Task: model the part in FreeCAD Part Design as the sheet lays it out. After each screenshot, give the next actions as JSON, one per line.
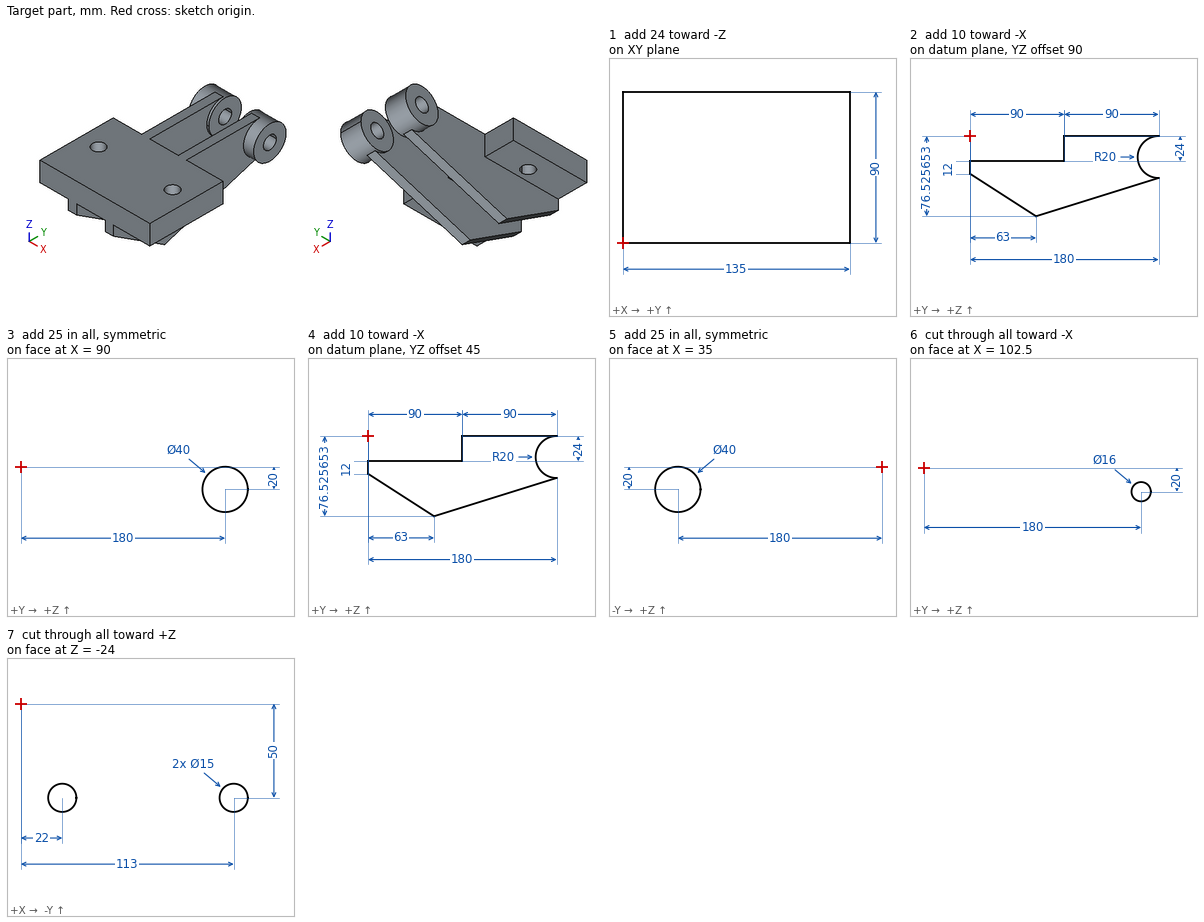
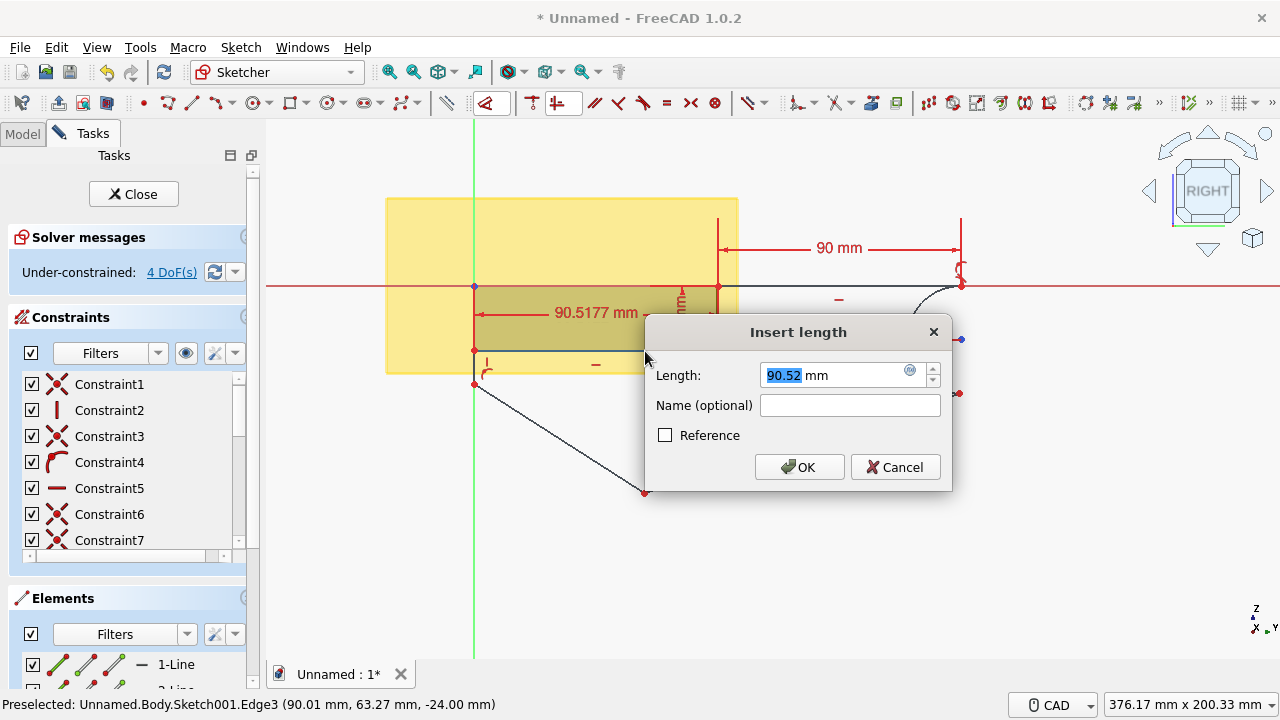
{"action": "type", "text": "90"}
{"action": "key", "text": "Return"}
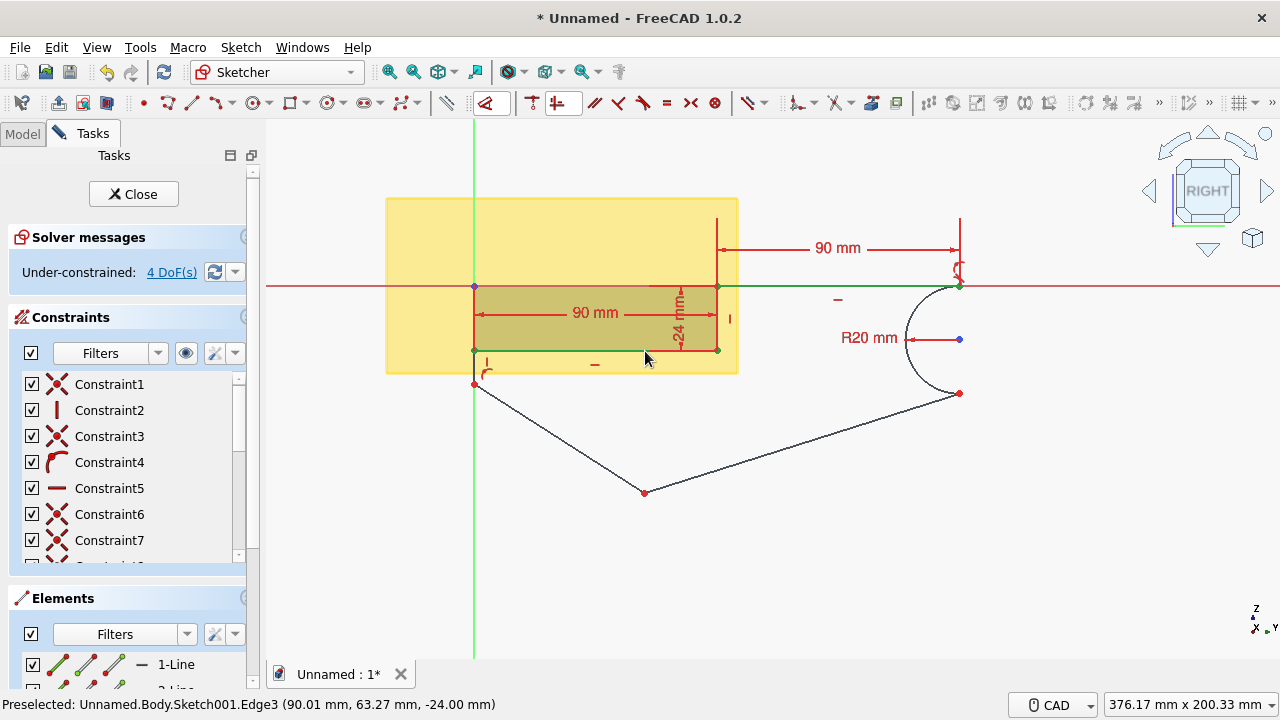
{"action": "scroll", "coordinate": [474, 361], "scroll_direction": "up", "scroll_amount": 2}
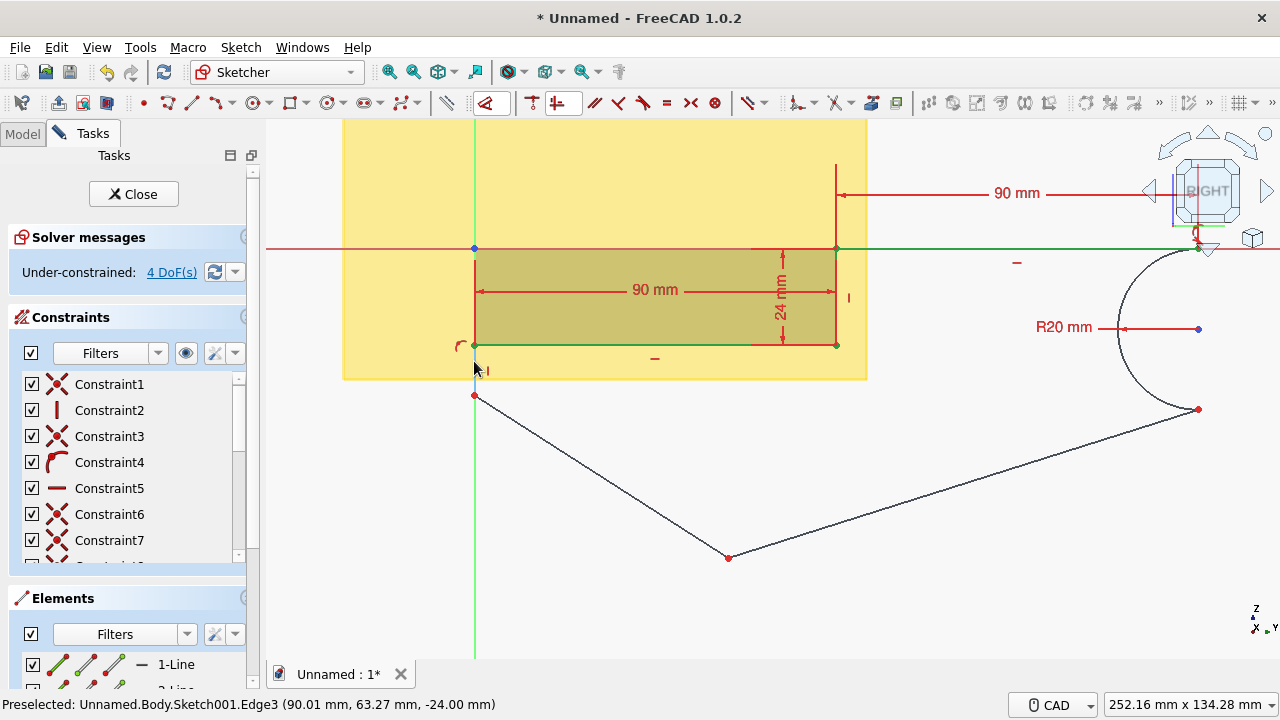
{"action": "left_click", "coordinate": [475, 360]}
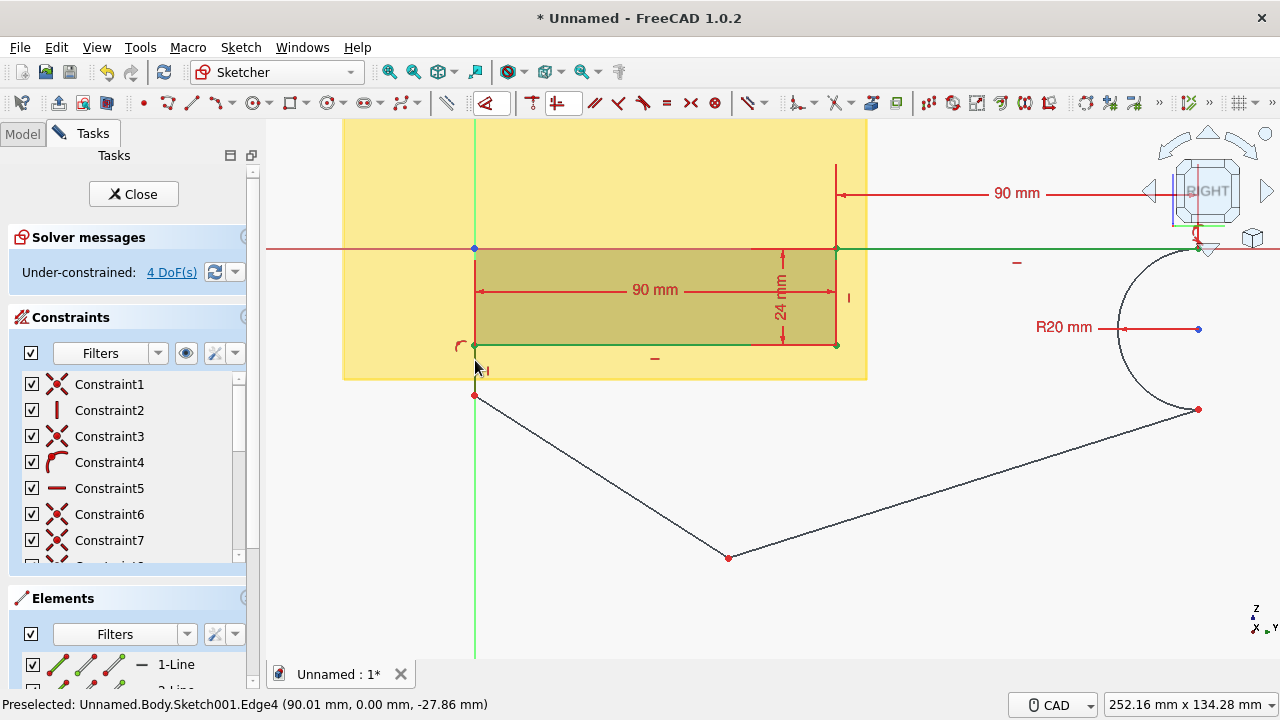
{"action": "key", "text": "i"}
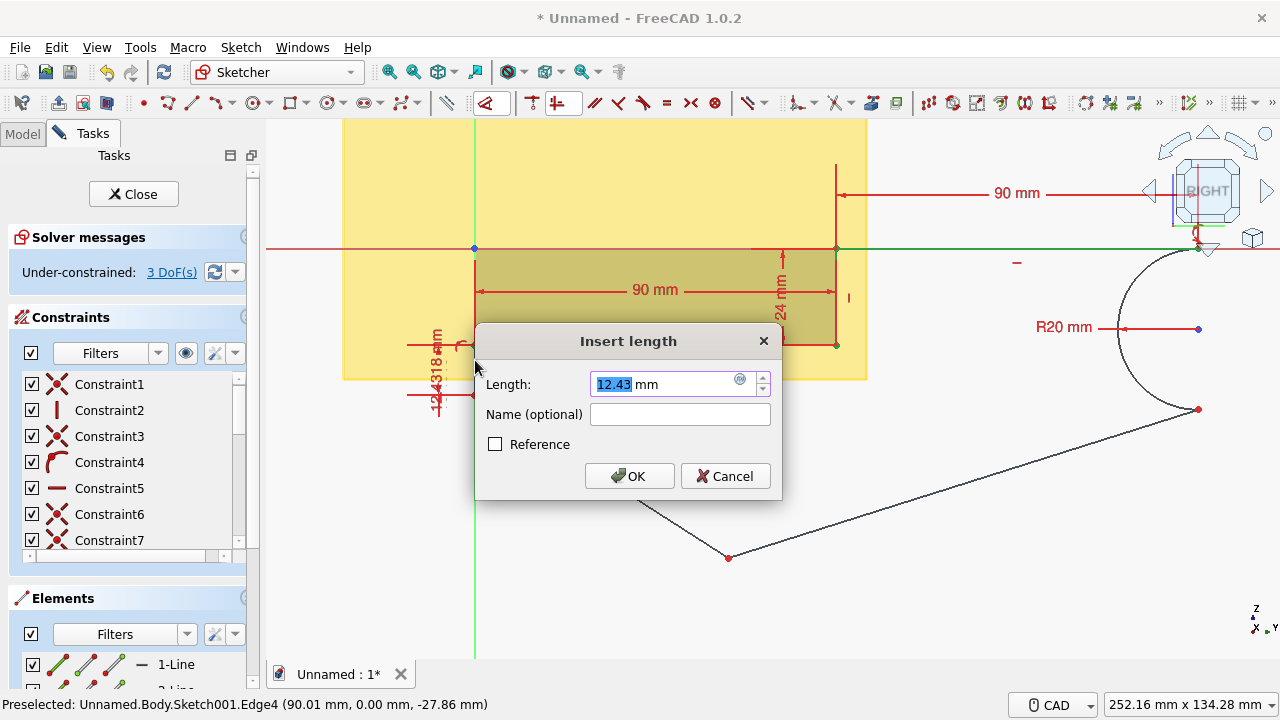
{"action": "type", "text": "12"}
{"action": "key", "text": "Return"}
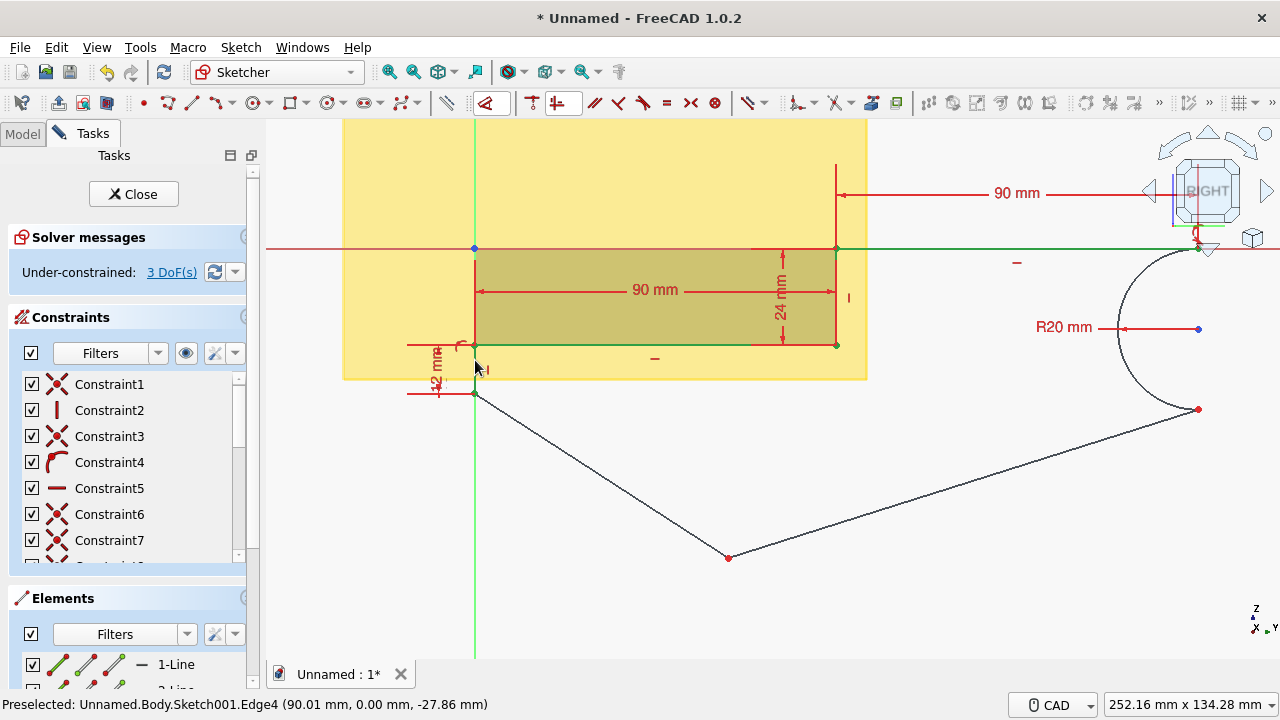
{"action": "left_click", "coordinate": [728, 558]}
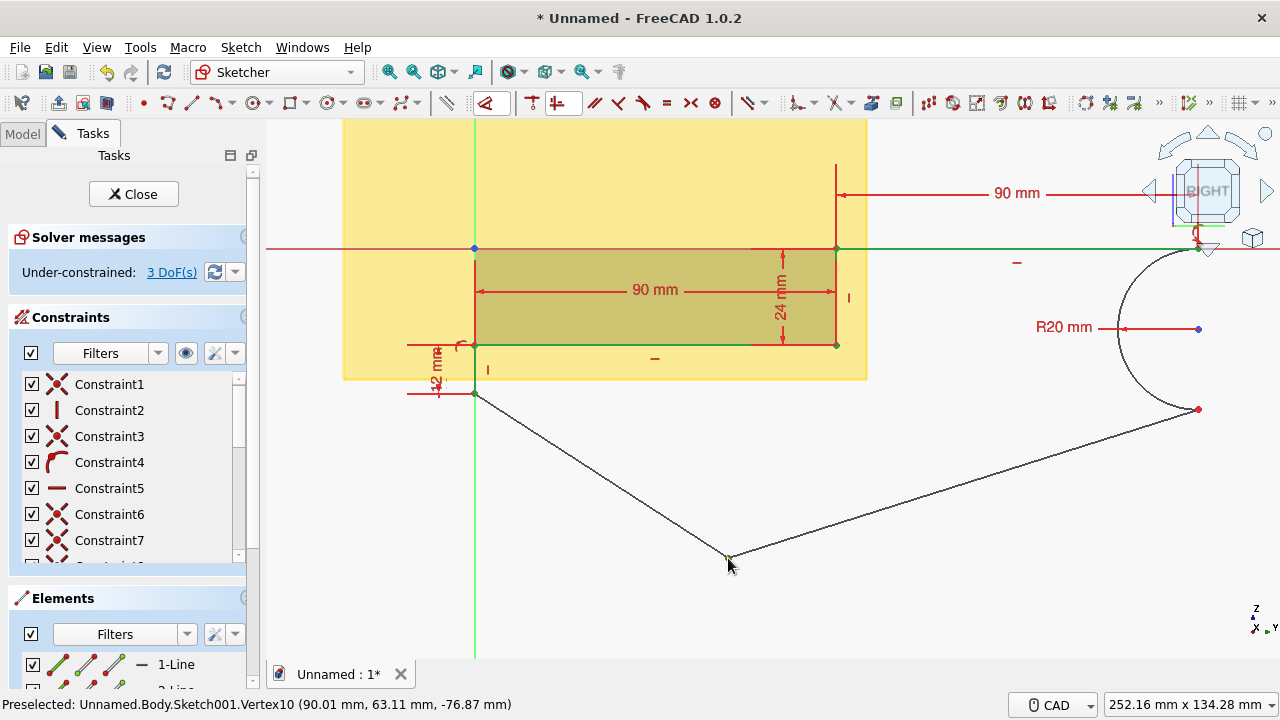
{"action": "key", "text": "l"}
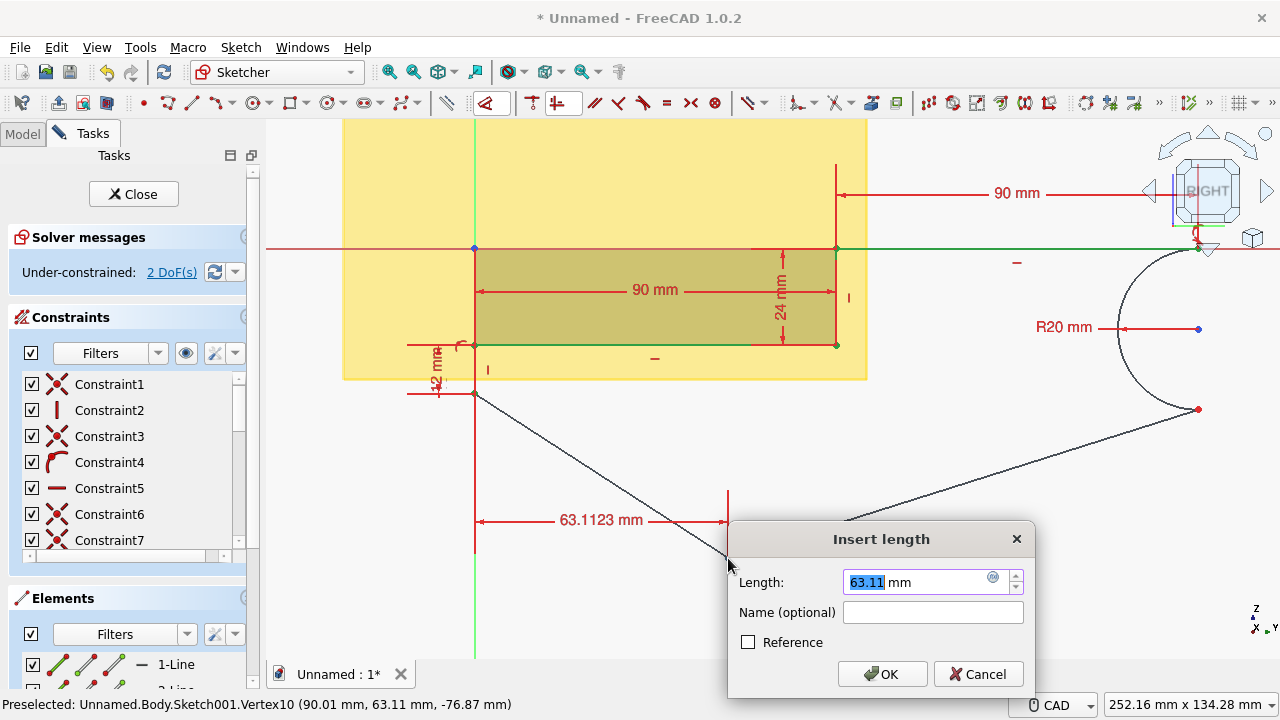
{"action": "type", "text": "63"}
{"action": "key", "text": "Return"}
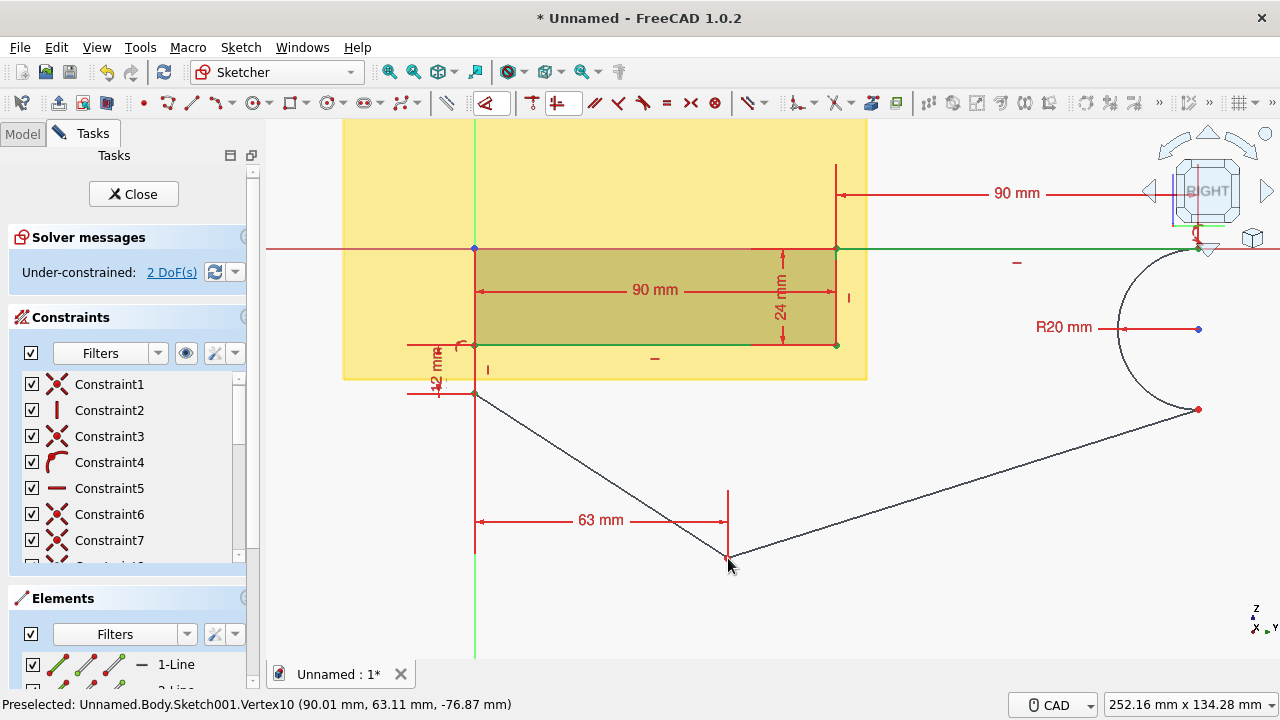
{"action": "scroll", "coordinate": [294, 327], "scroll_direction": "down", "scroll_amount": 1}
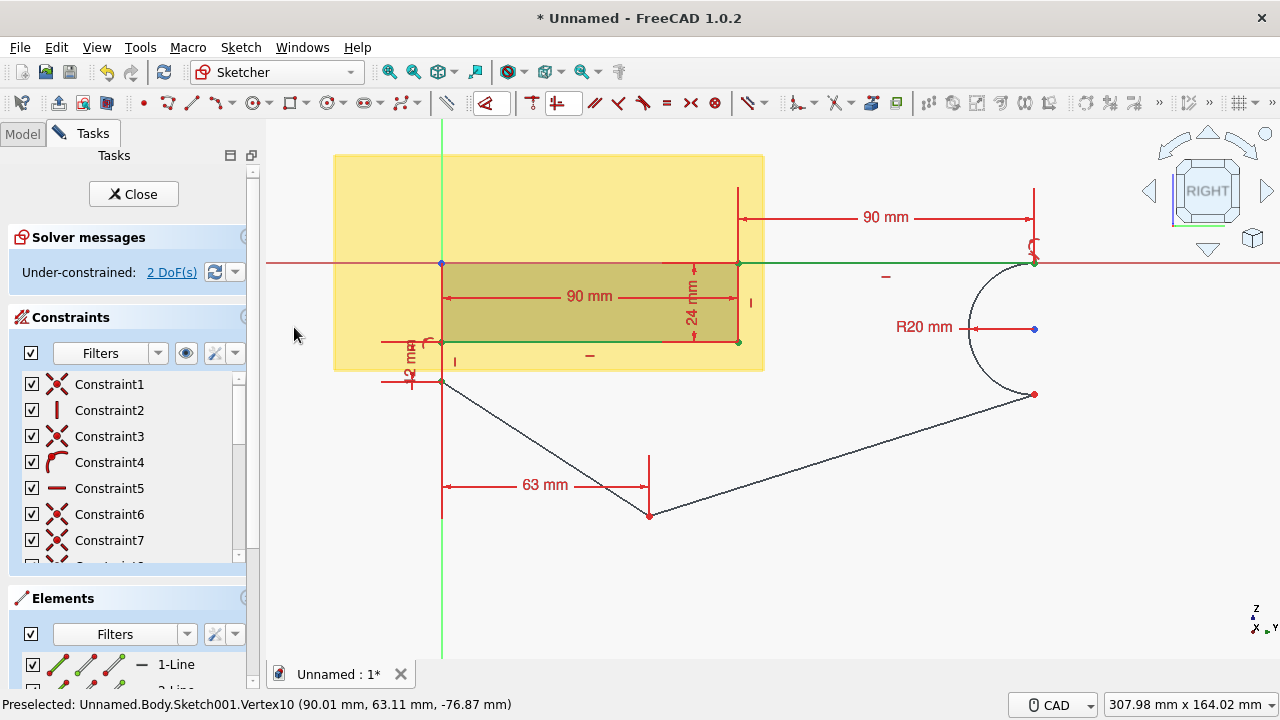
{"action": "left_click", "coordinate": [1034, 395]}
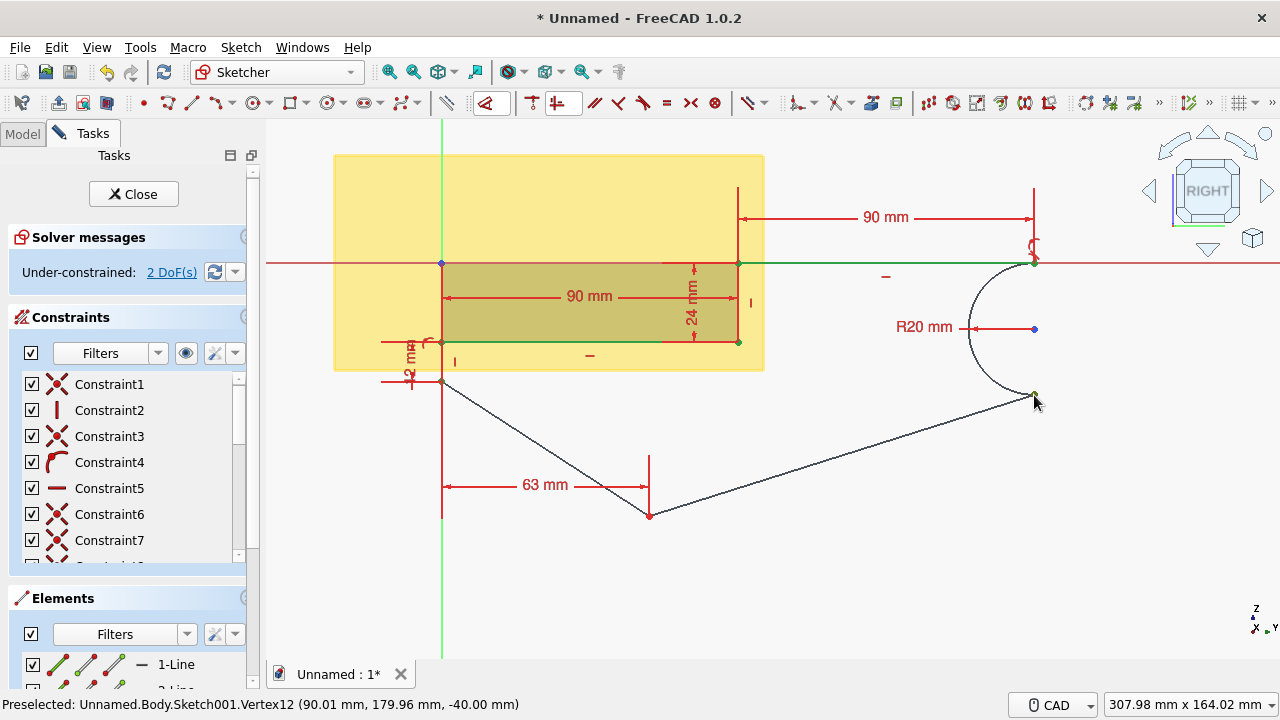
{"action": "left_click", "coordinate": [504, 104]}